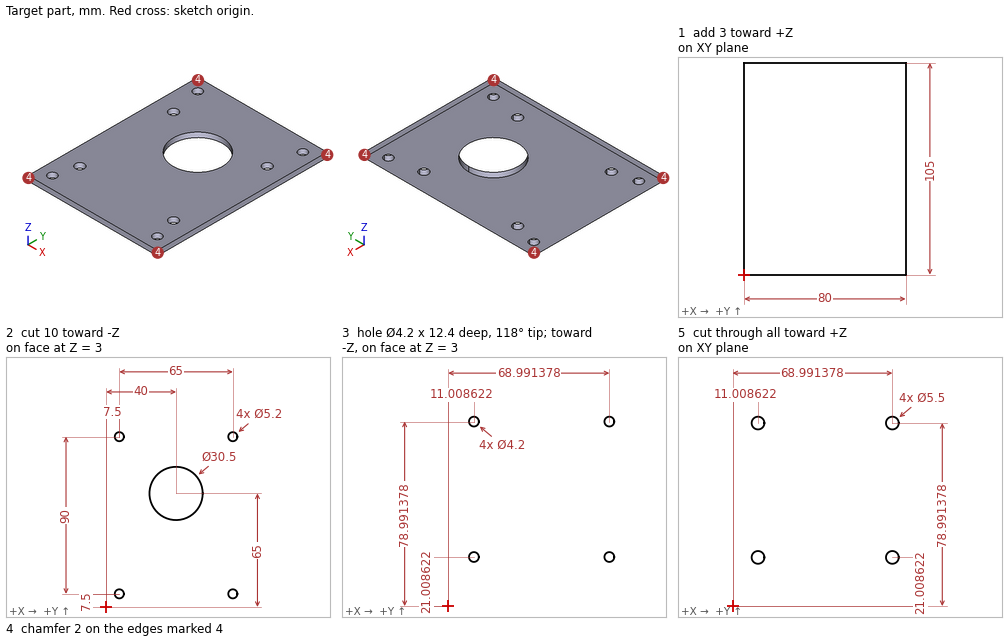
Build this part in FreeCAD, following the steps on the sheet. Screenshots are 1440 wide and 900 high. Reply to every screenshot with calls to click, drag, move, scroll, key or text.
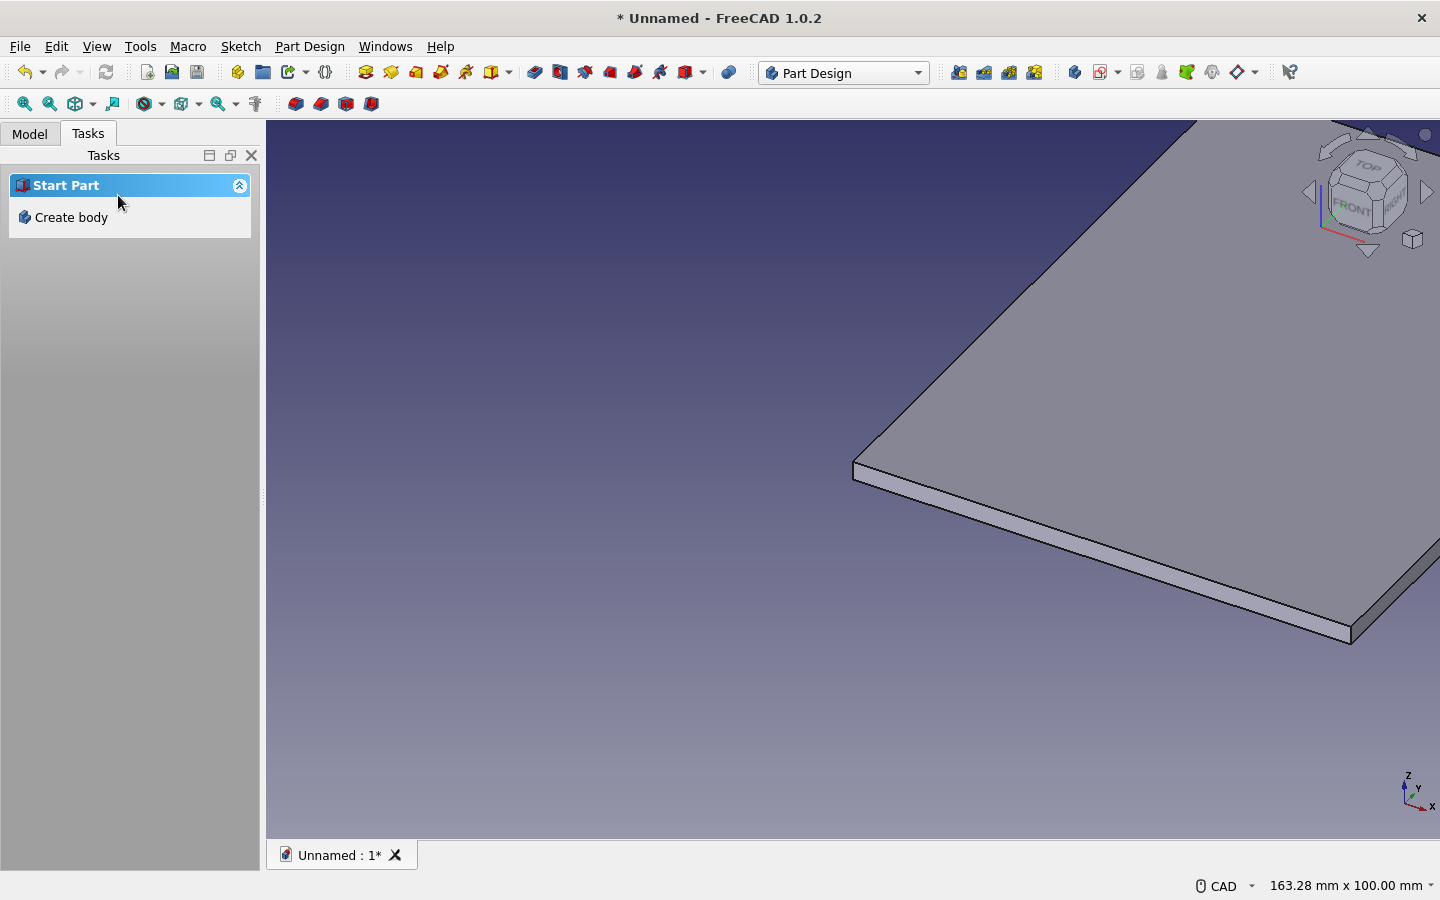
click(25, 104)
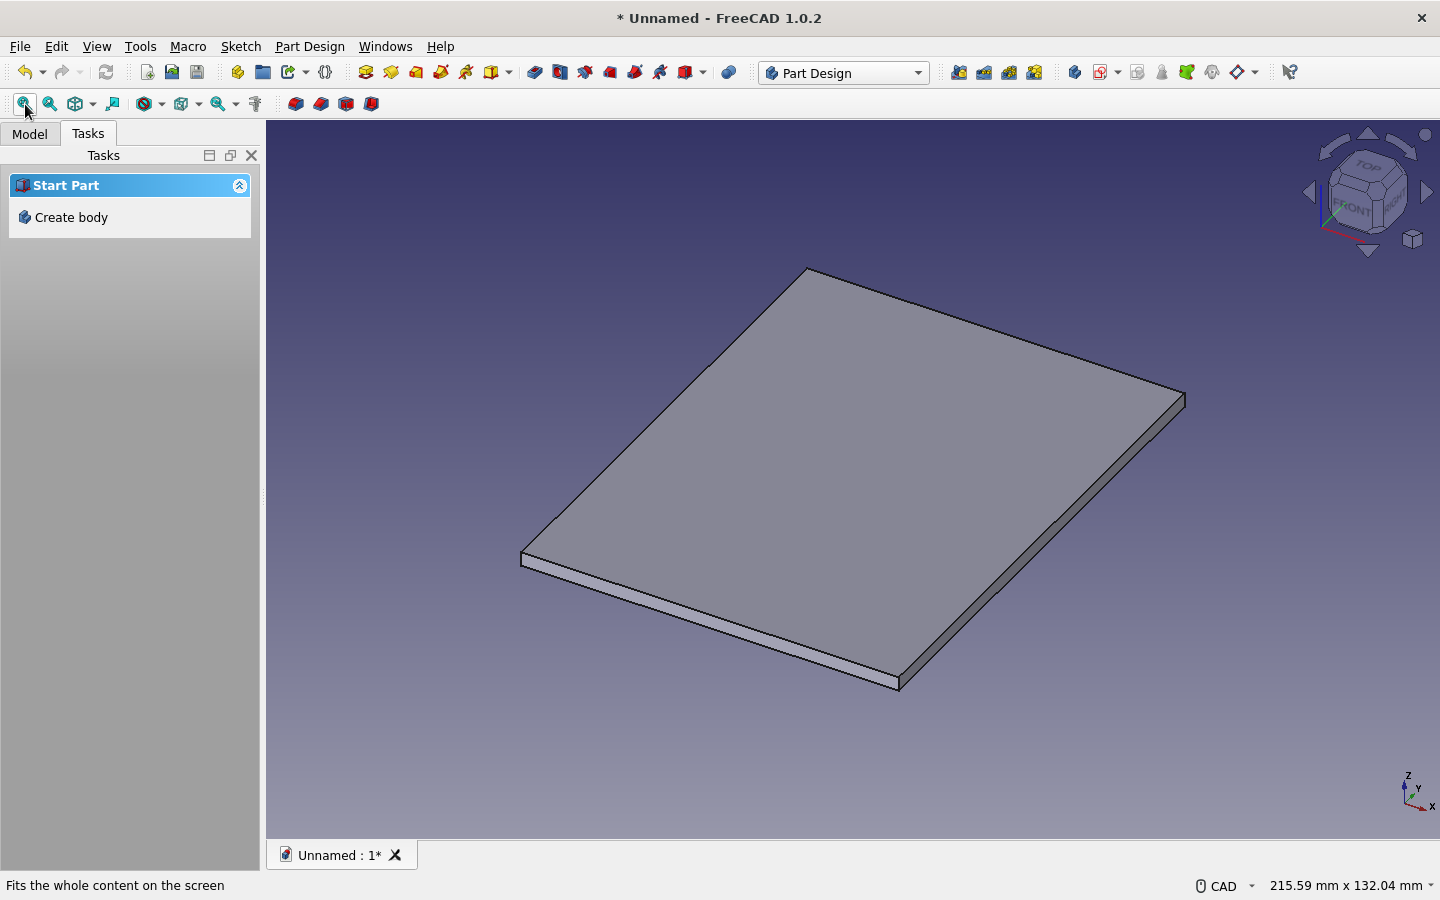
click(853, 472)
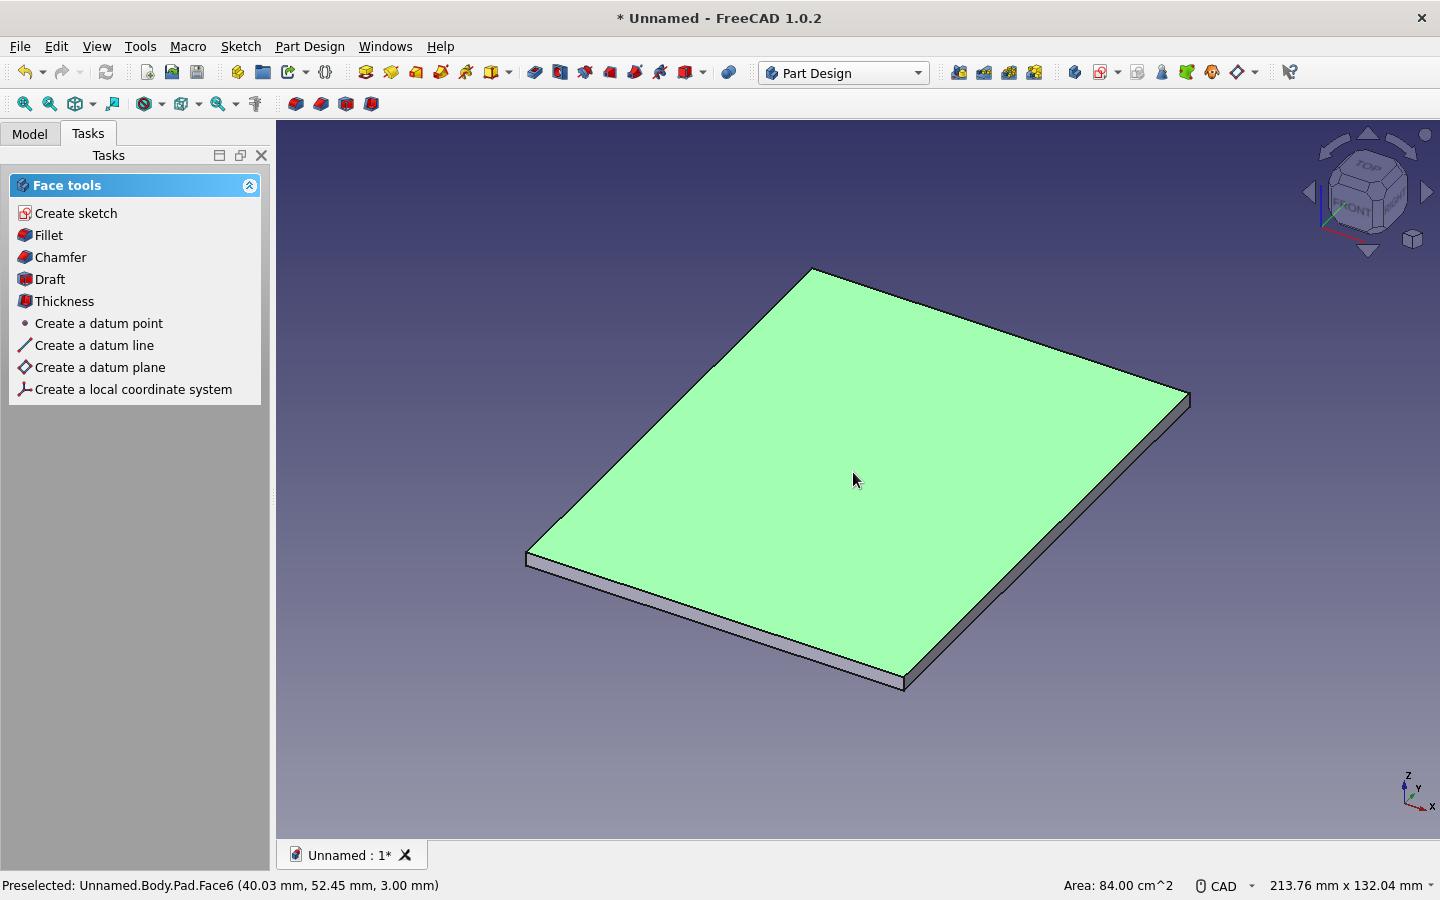
click(1100, 72)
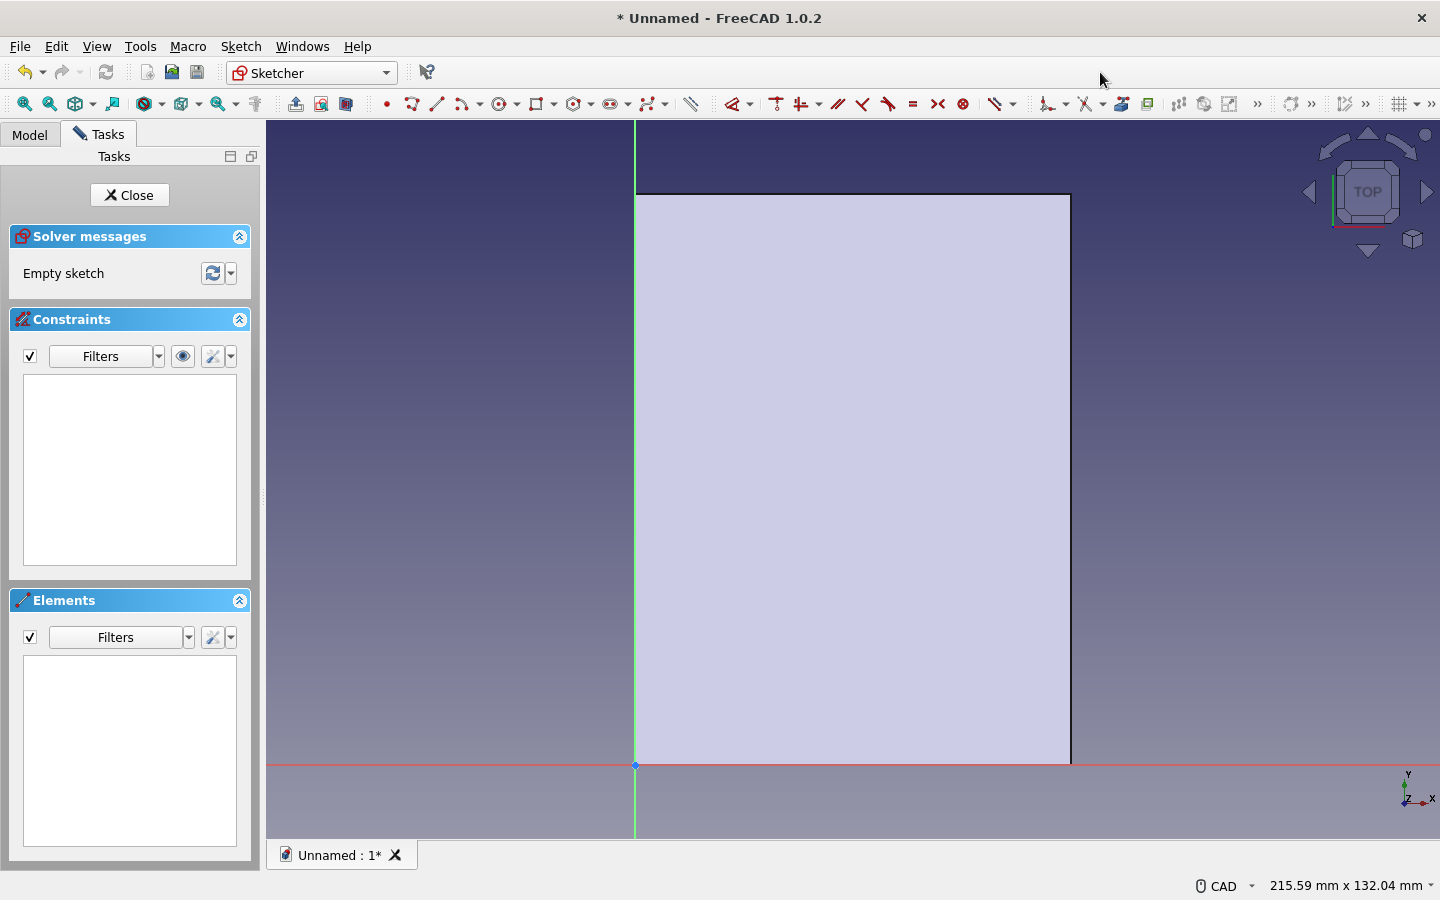
click(498, 104)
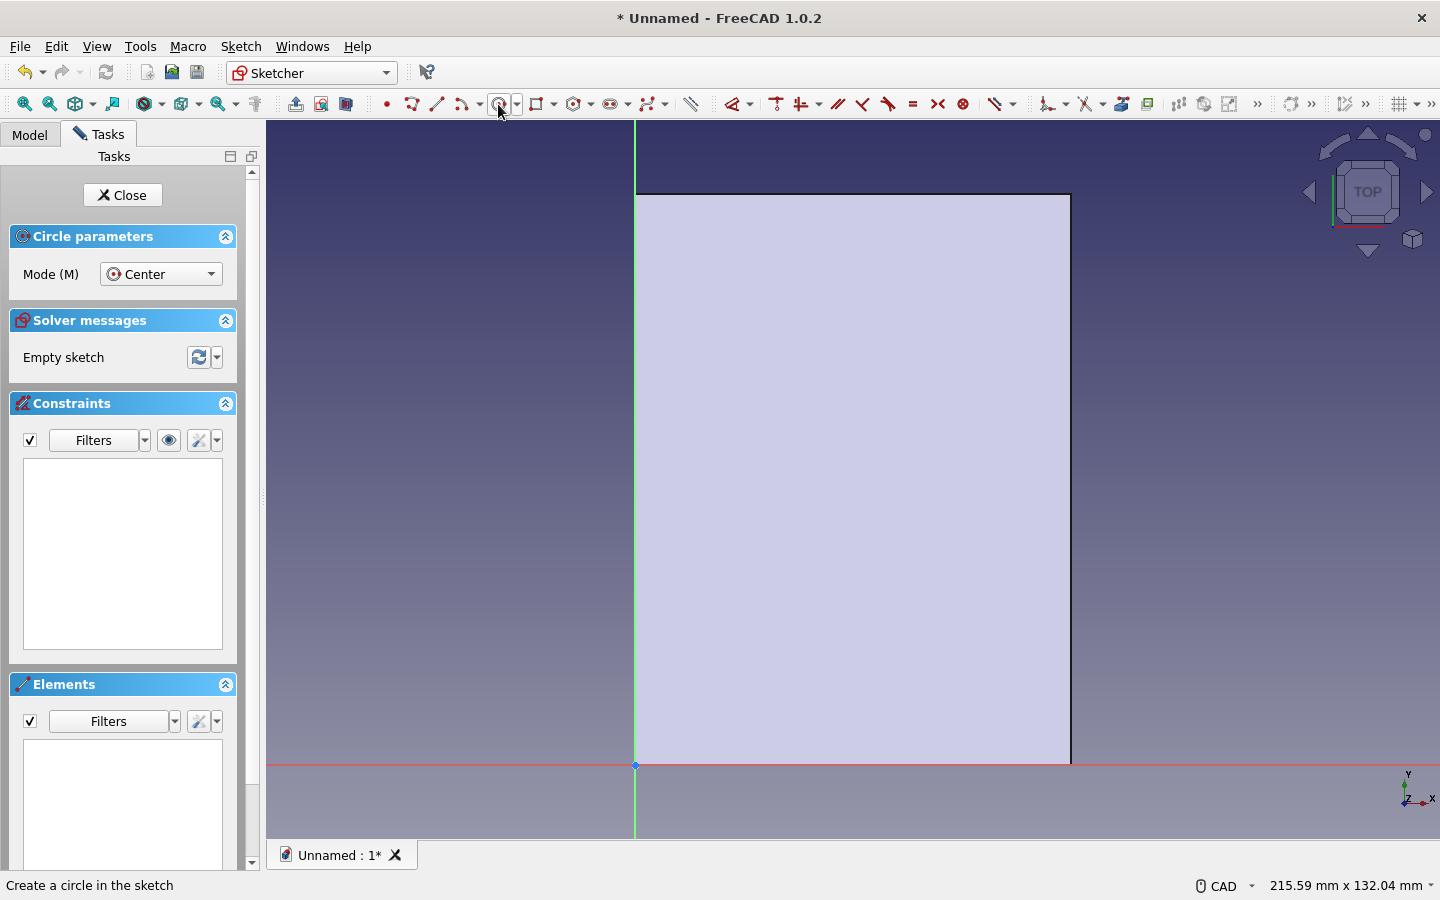
scroll(676, 234, up, 3)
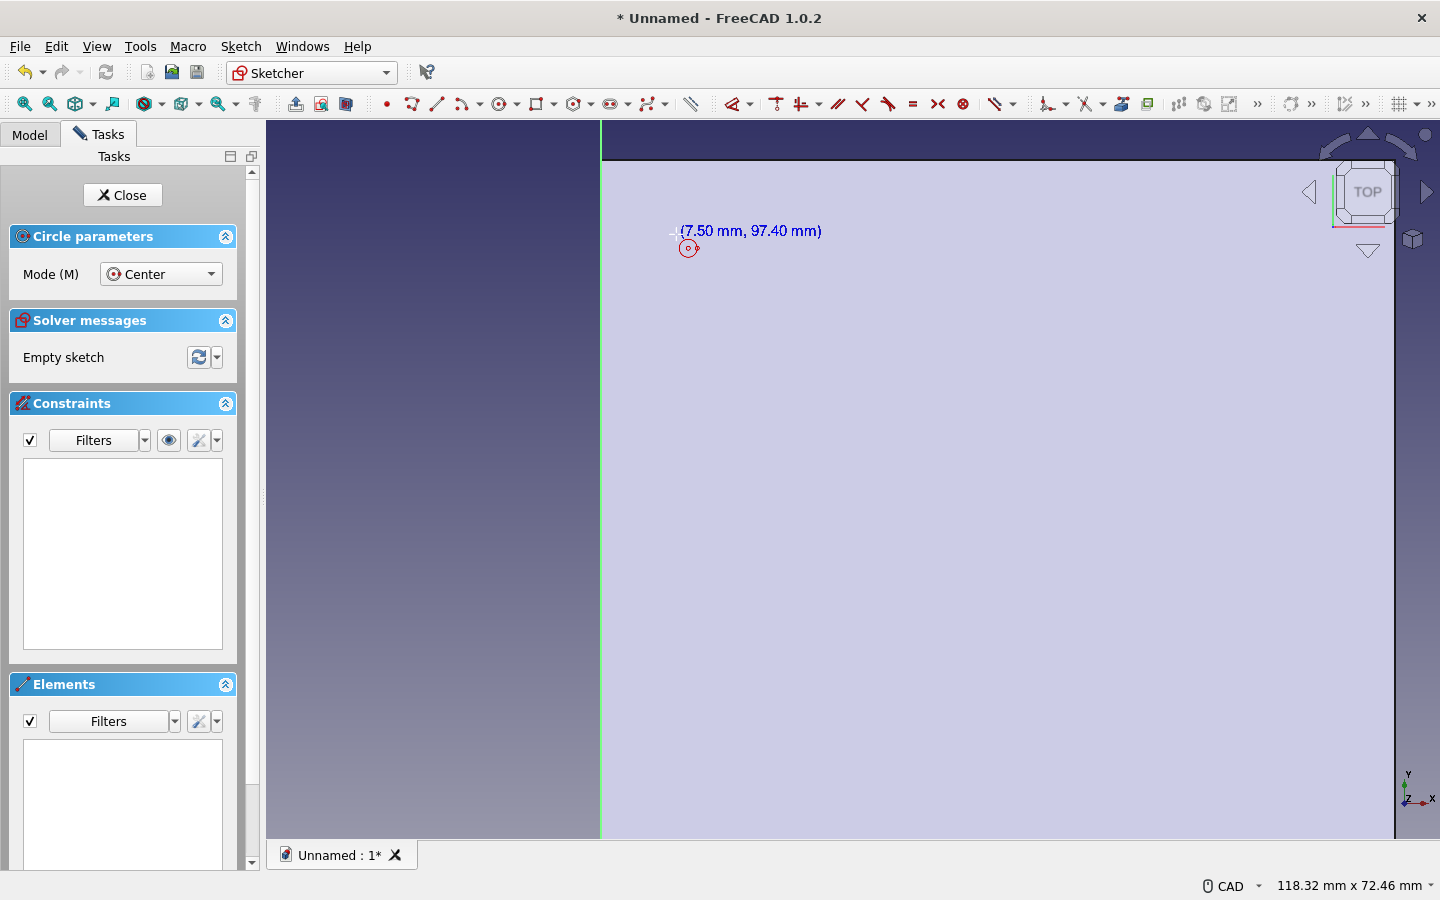
click(676, 235)
click(694, 216)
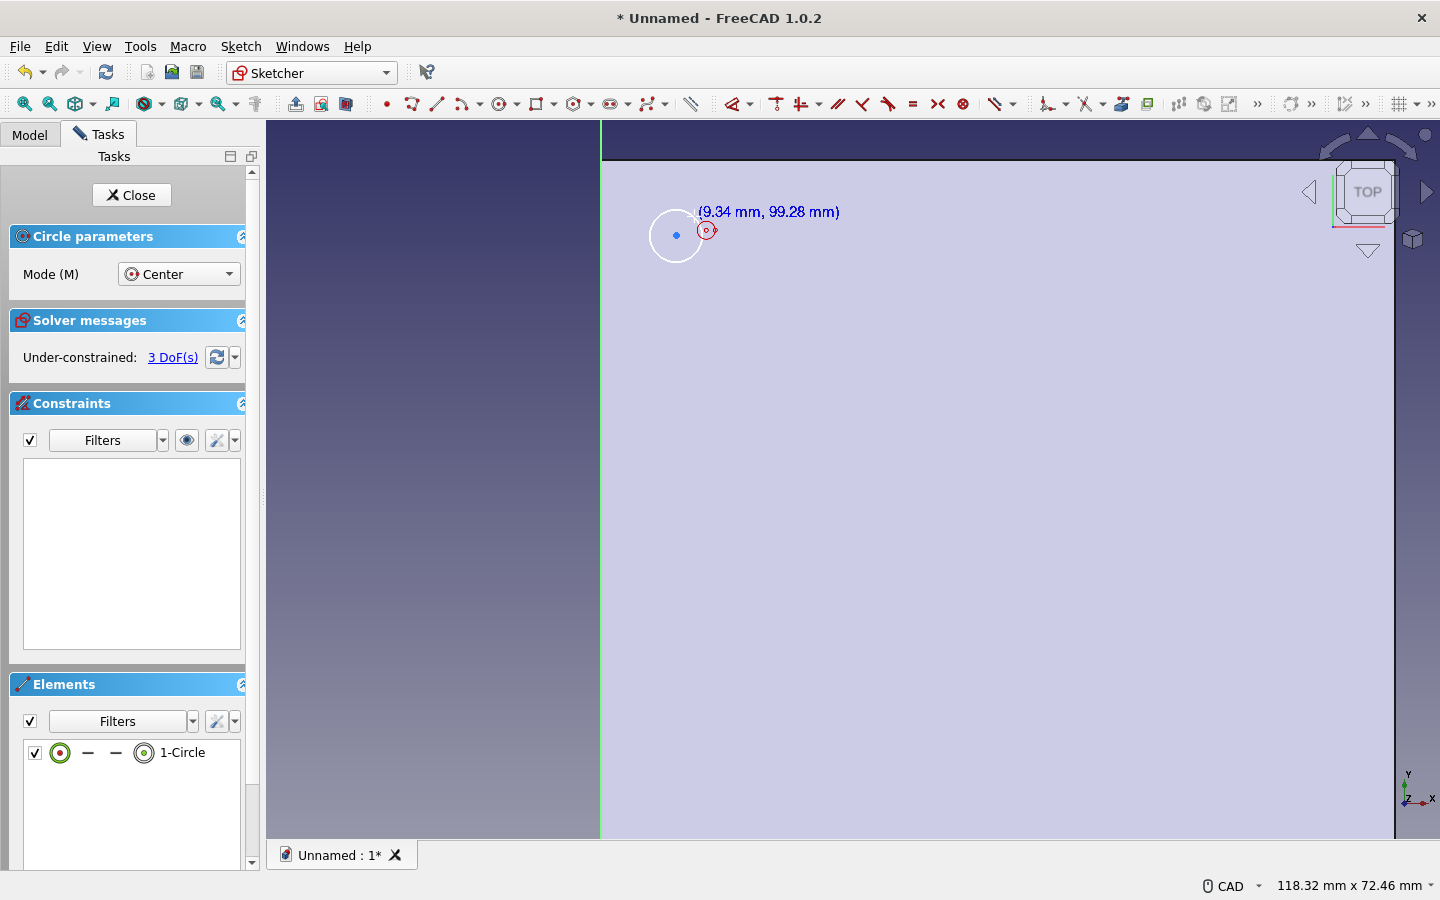
scroll(630, 295, down, 4)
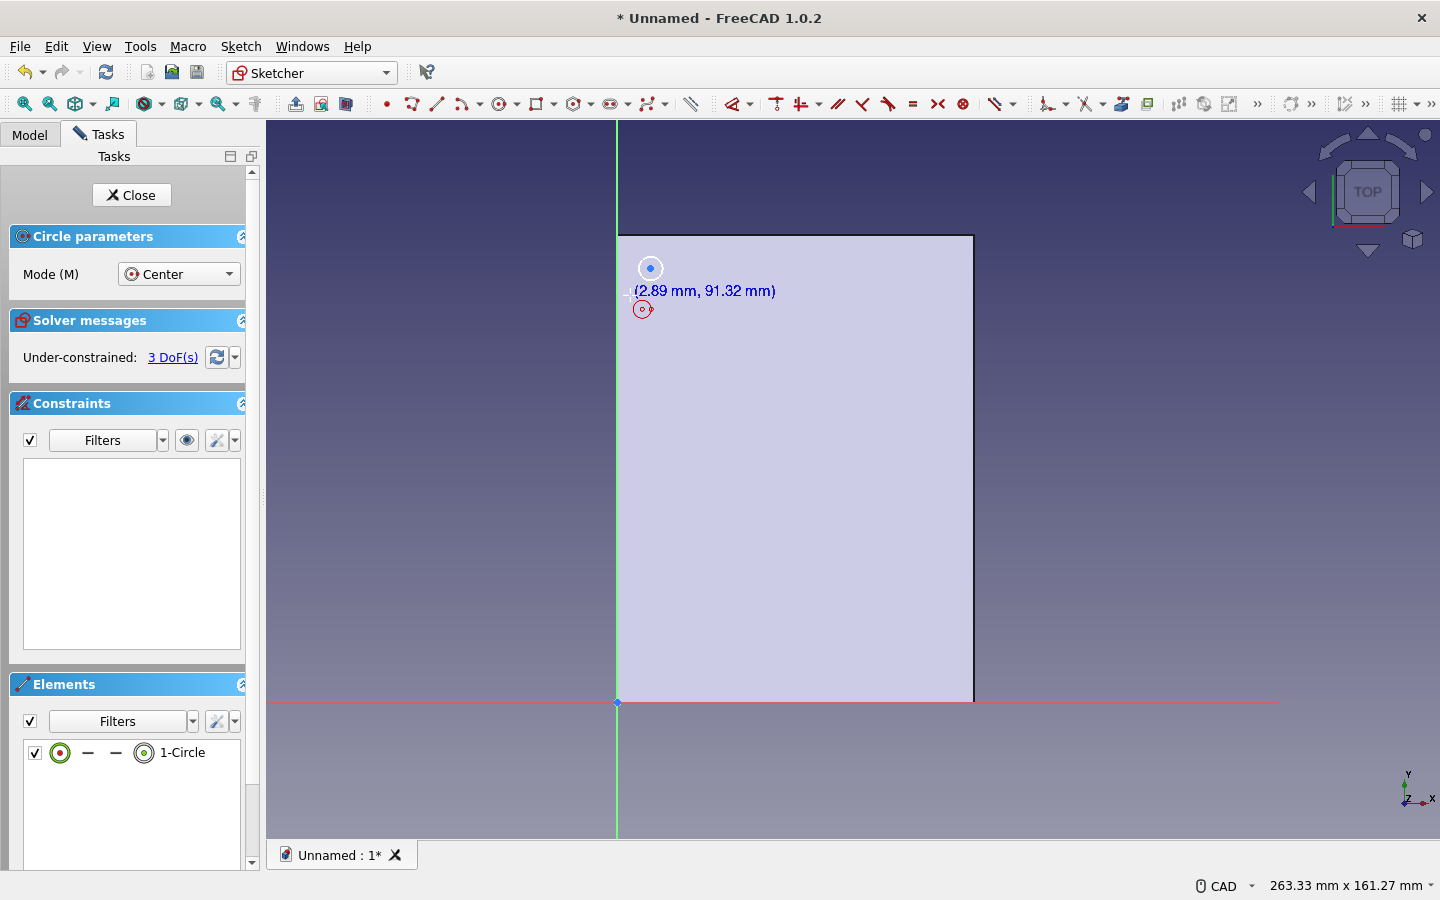
scroll(941, 268, up, 4)